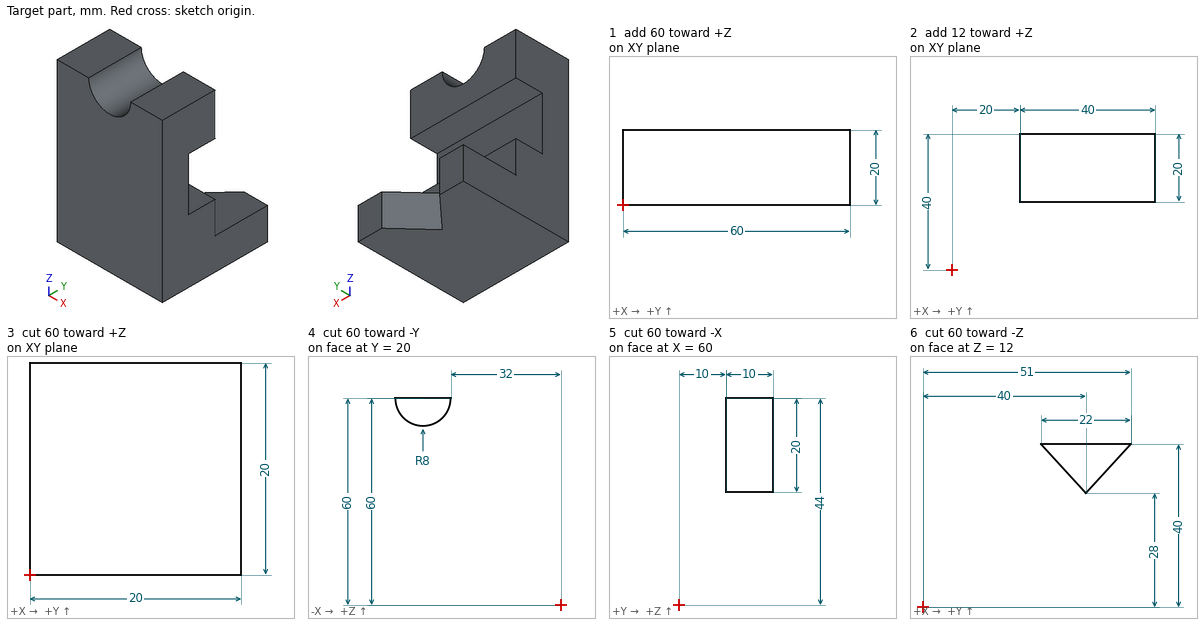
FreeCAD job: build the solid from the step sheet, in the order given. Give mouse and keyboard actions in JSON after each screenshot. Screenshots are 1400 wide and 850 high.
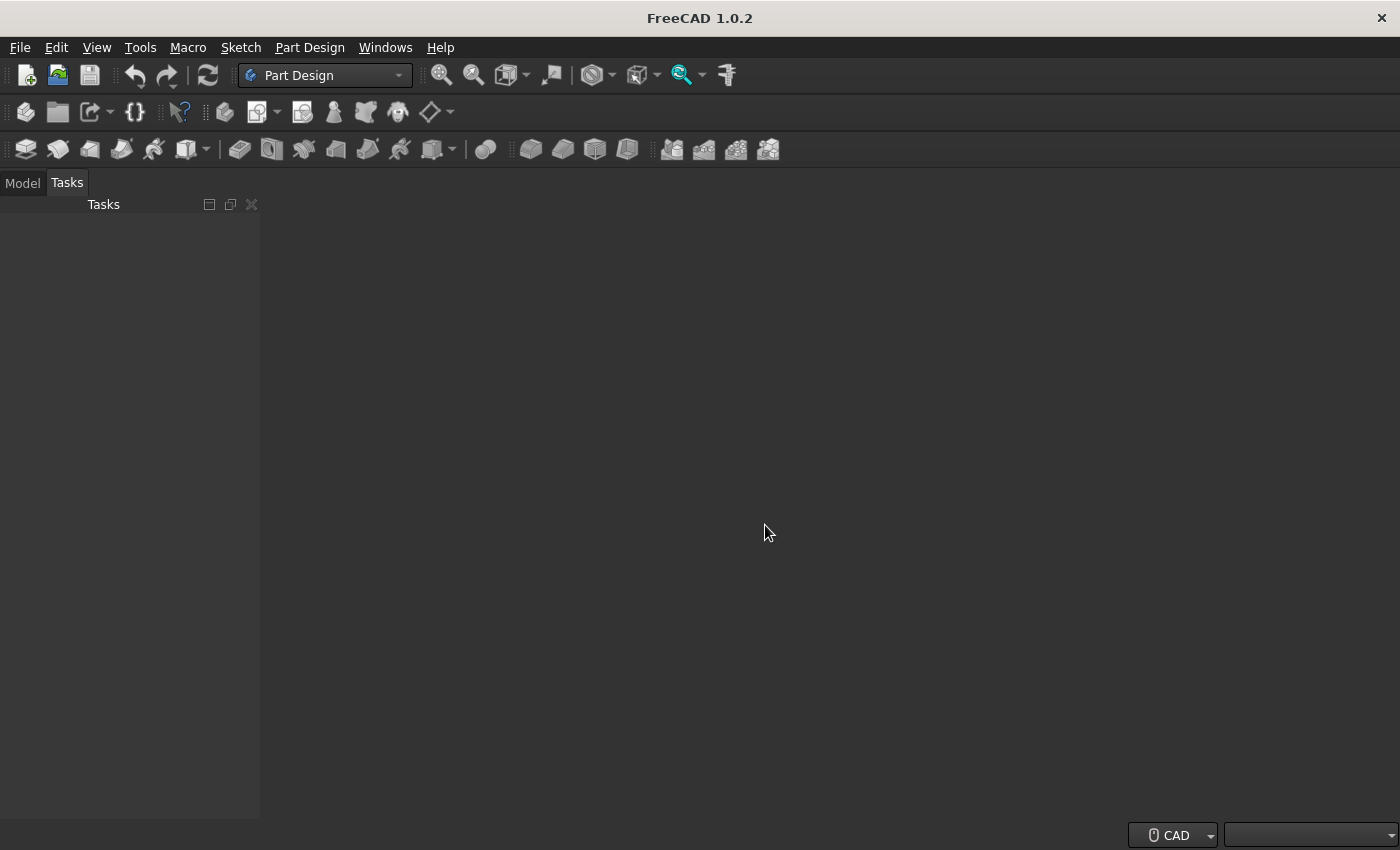
{"action": "left_click", "coordinate": [26, 76]}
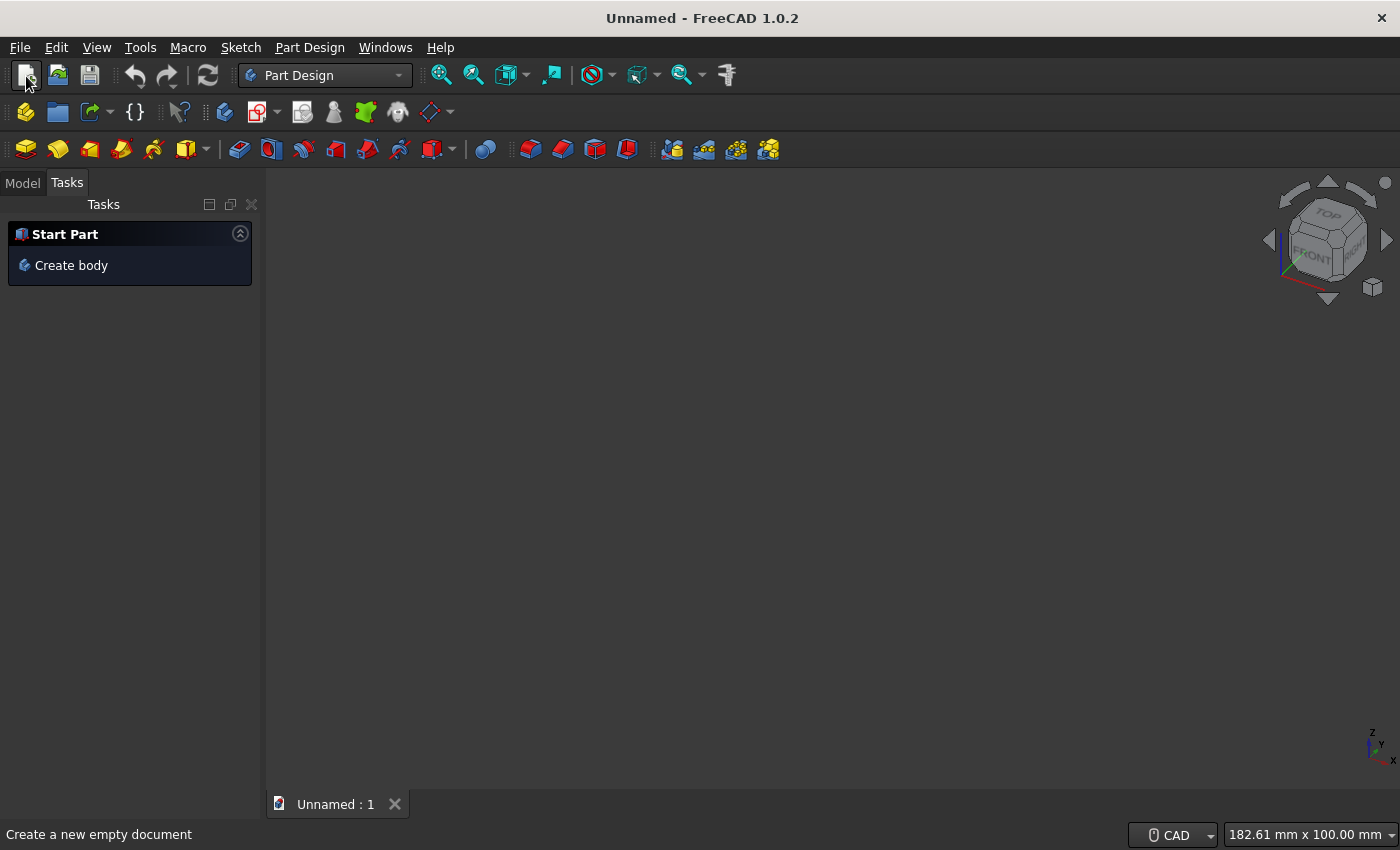
{"action": "left_click", "coordinate": [258, 112]}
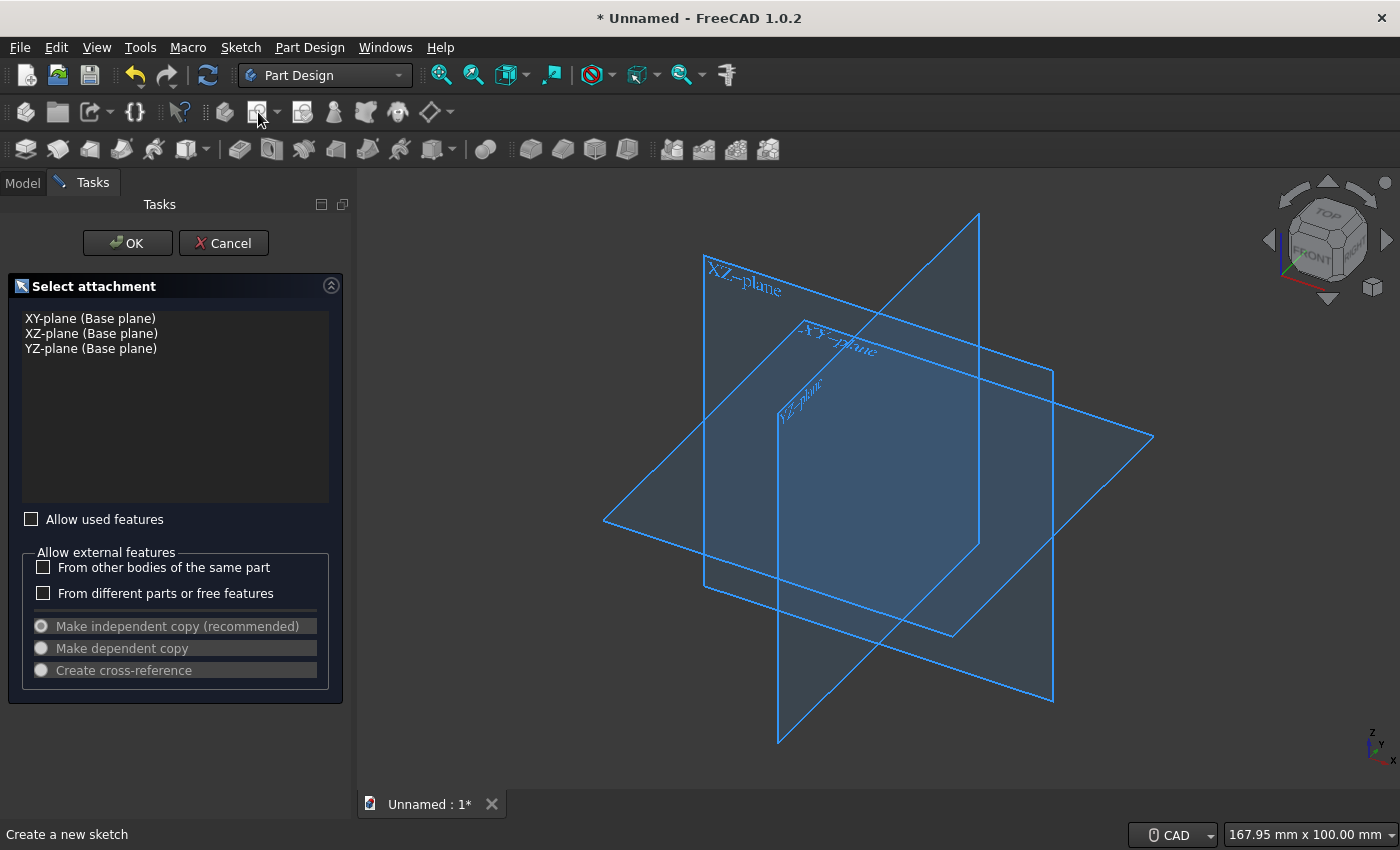
{"action": "left_click", "coordinate": [82, 318]}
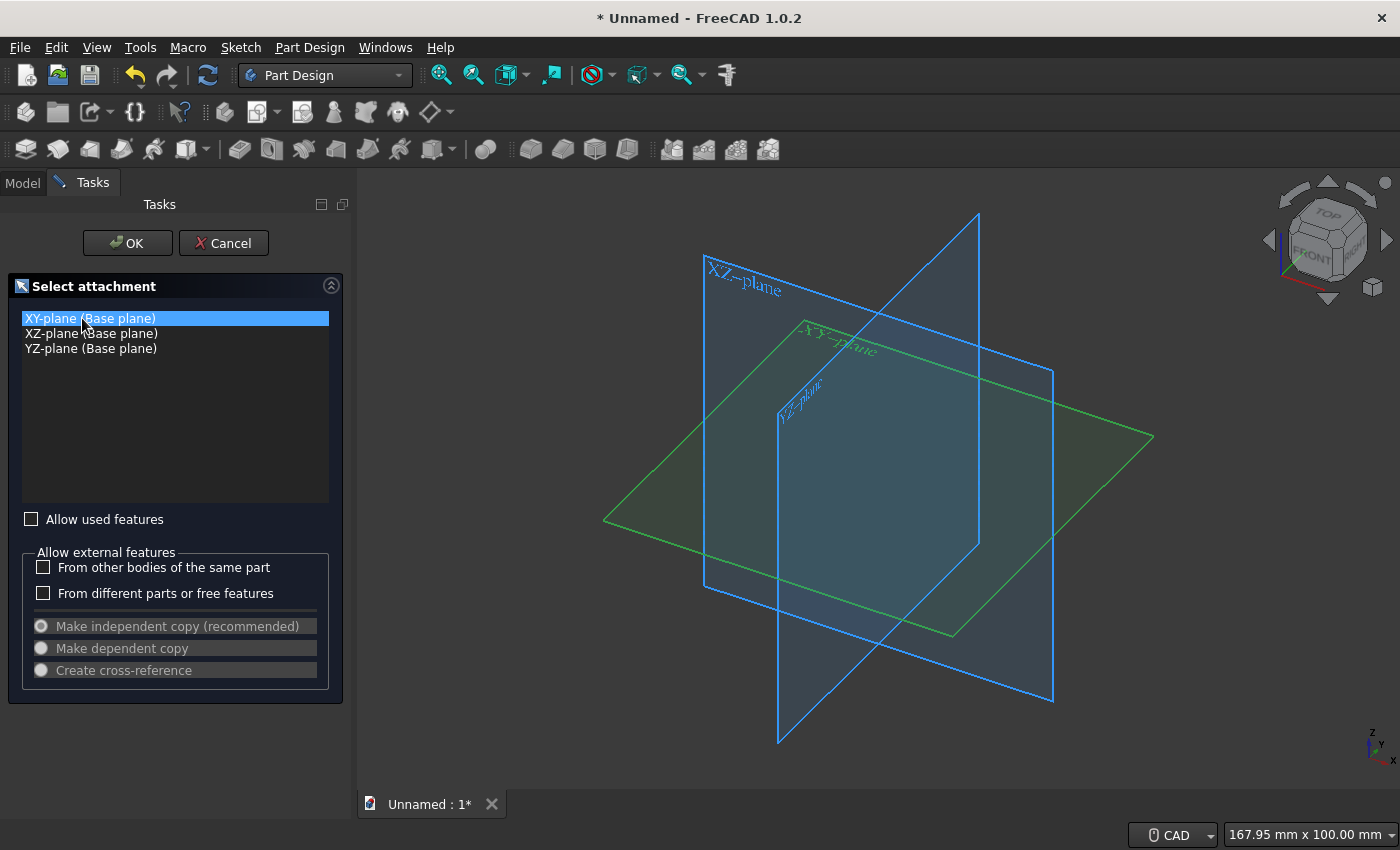
{"action": "left_click", "coordinate": [128, 243]}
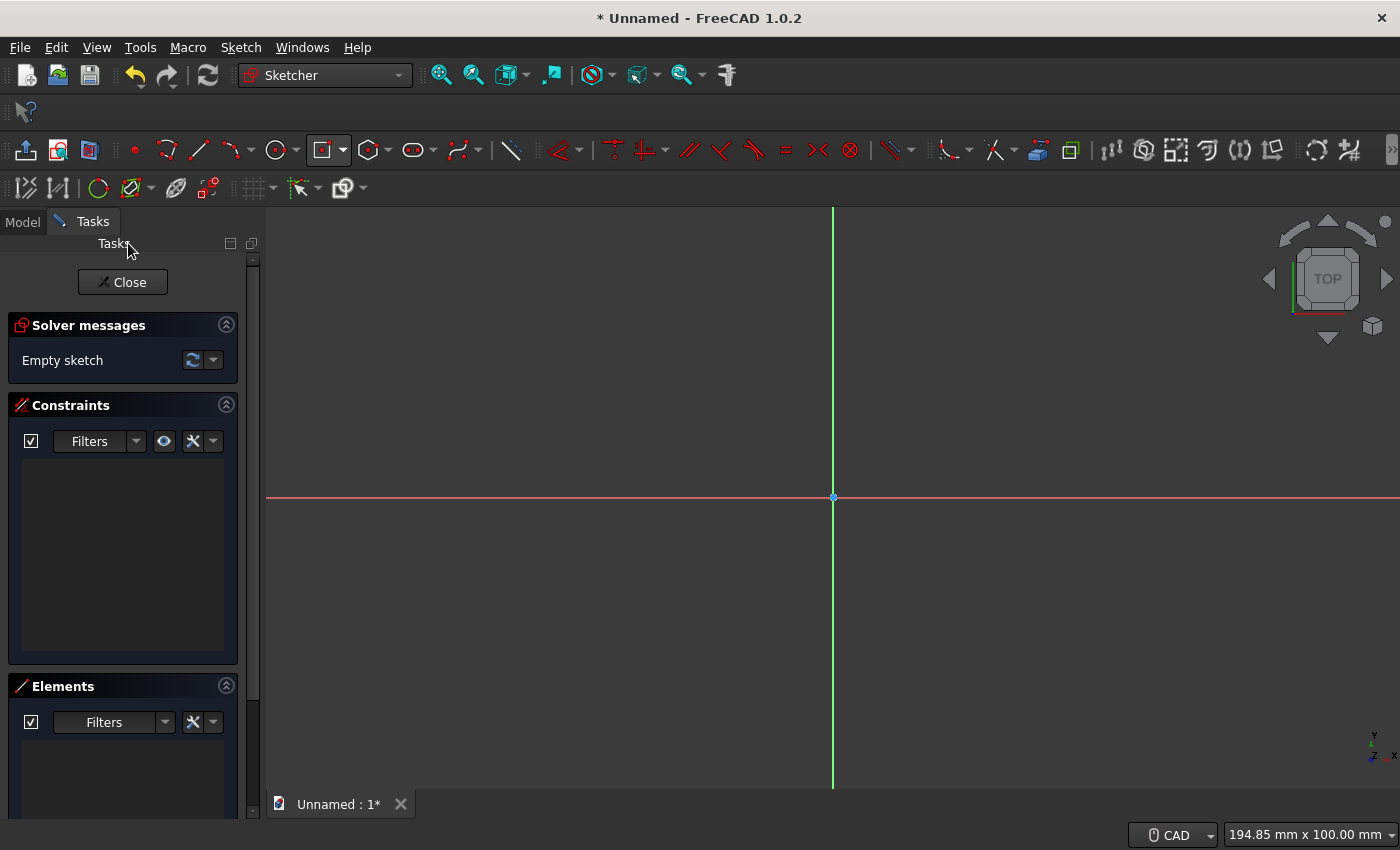
{"action": "scroll", "coordinate": [1235, 369], "scroll_direction": "up", "scroll_amount": 3}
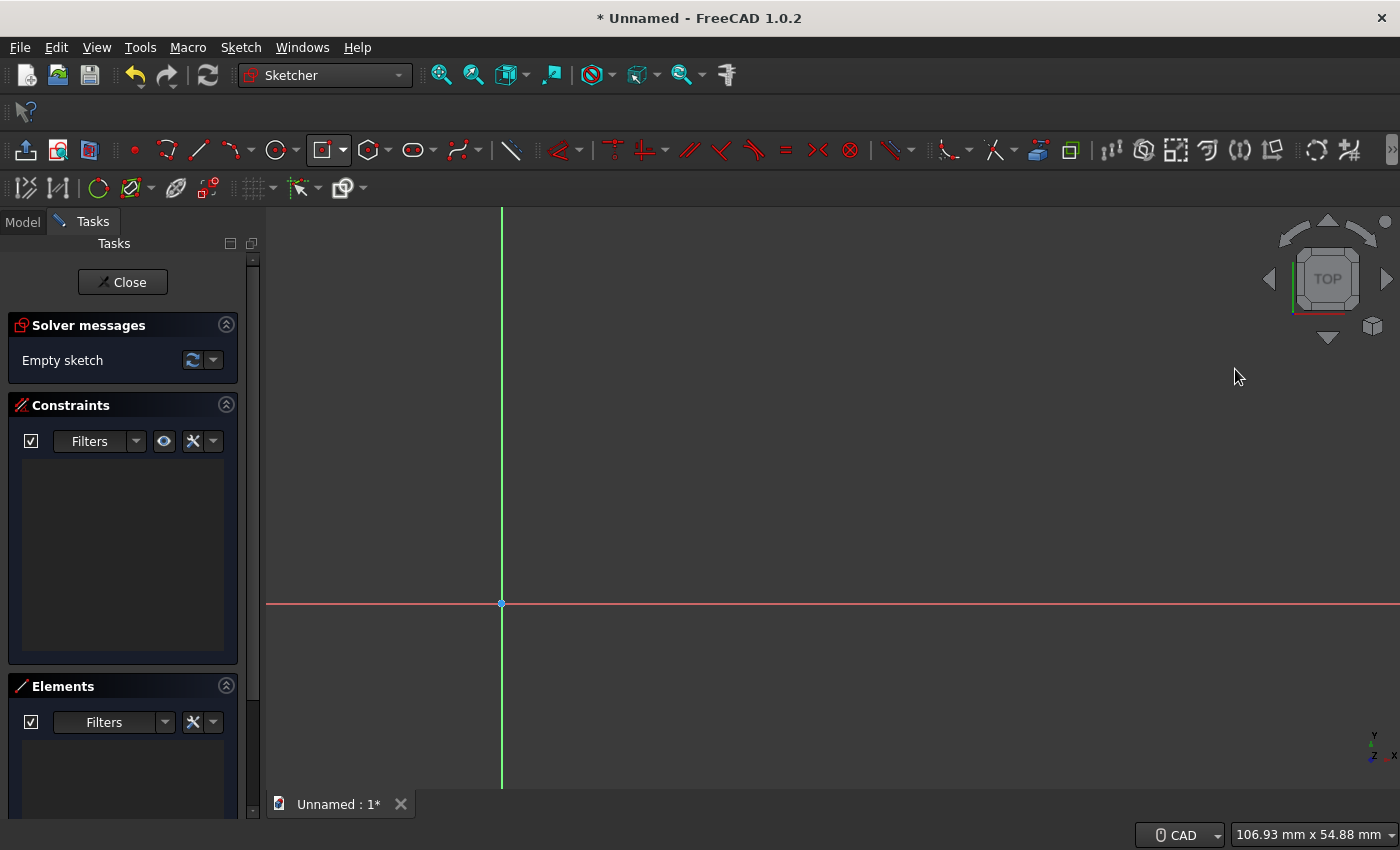
{"action": "key", "text": "g r"}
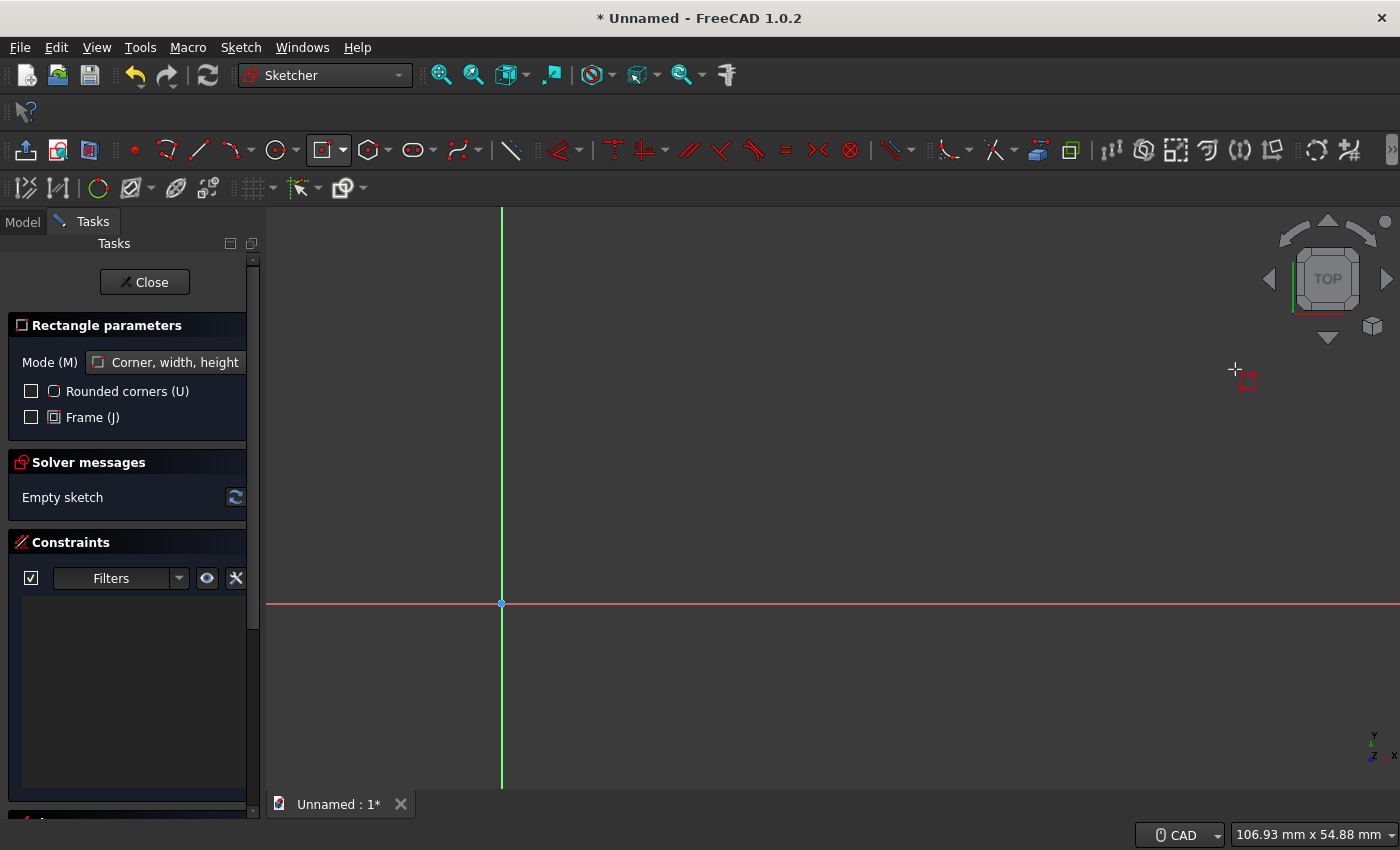
{"action": "left_click", "coordinate": [502, 604]}
{"action": "mouse_move", "coordinate": [1138, 392]}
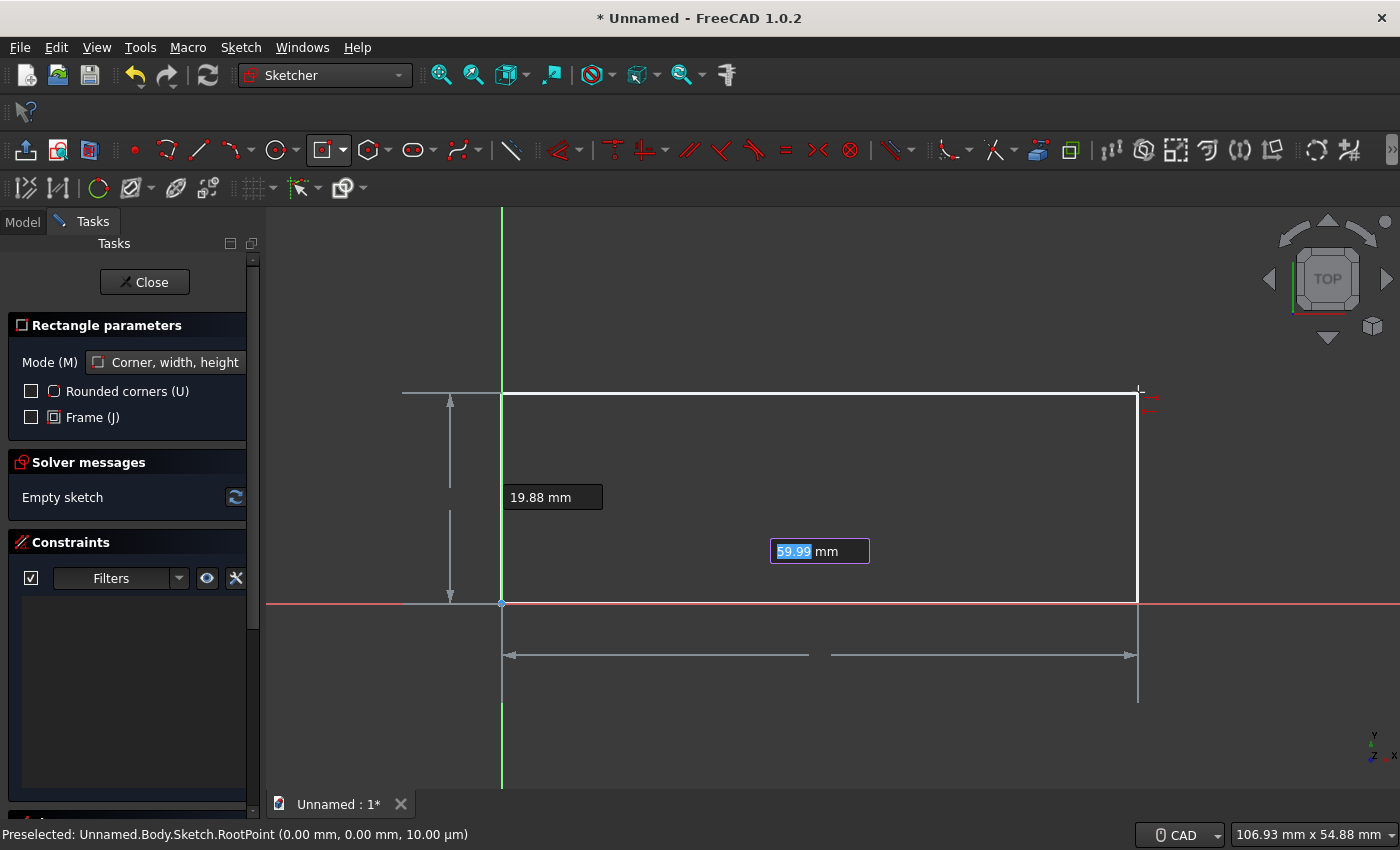
{"action": "type", "text": "60"}
{"action": "key", "text": "Tab"}
{"action": "type", "text": "20"}
{"action": "key", "text": "Return"}
{"action": "key", "text": "Escape"}